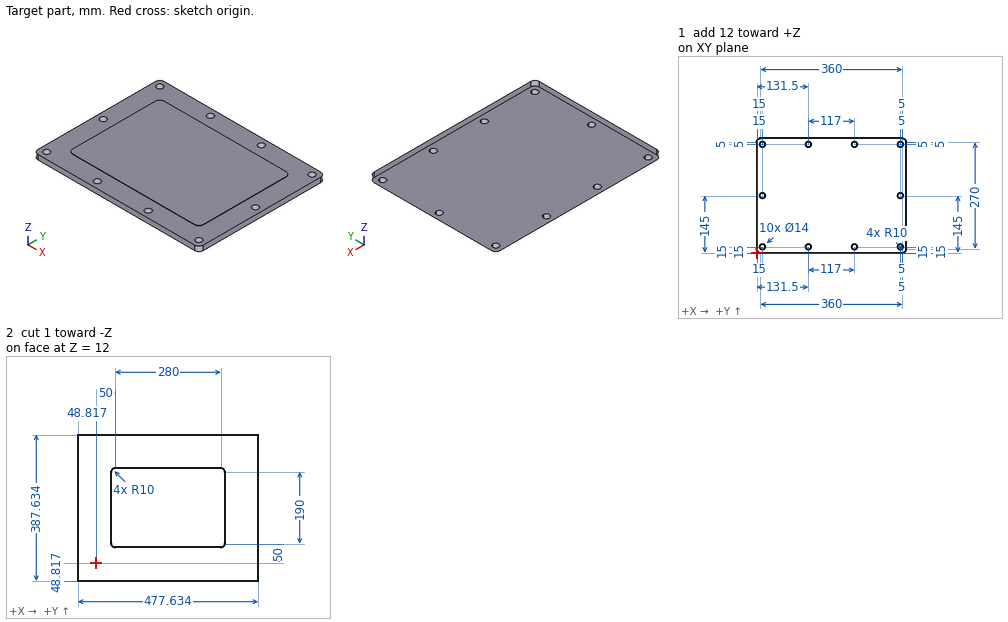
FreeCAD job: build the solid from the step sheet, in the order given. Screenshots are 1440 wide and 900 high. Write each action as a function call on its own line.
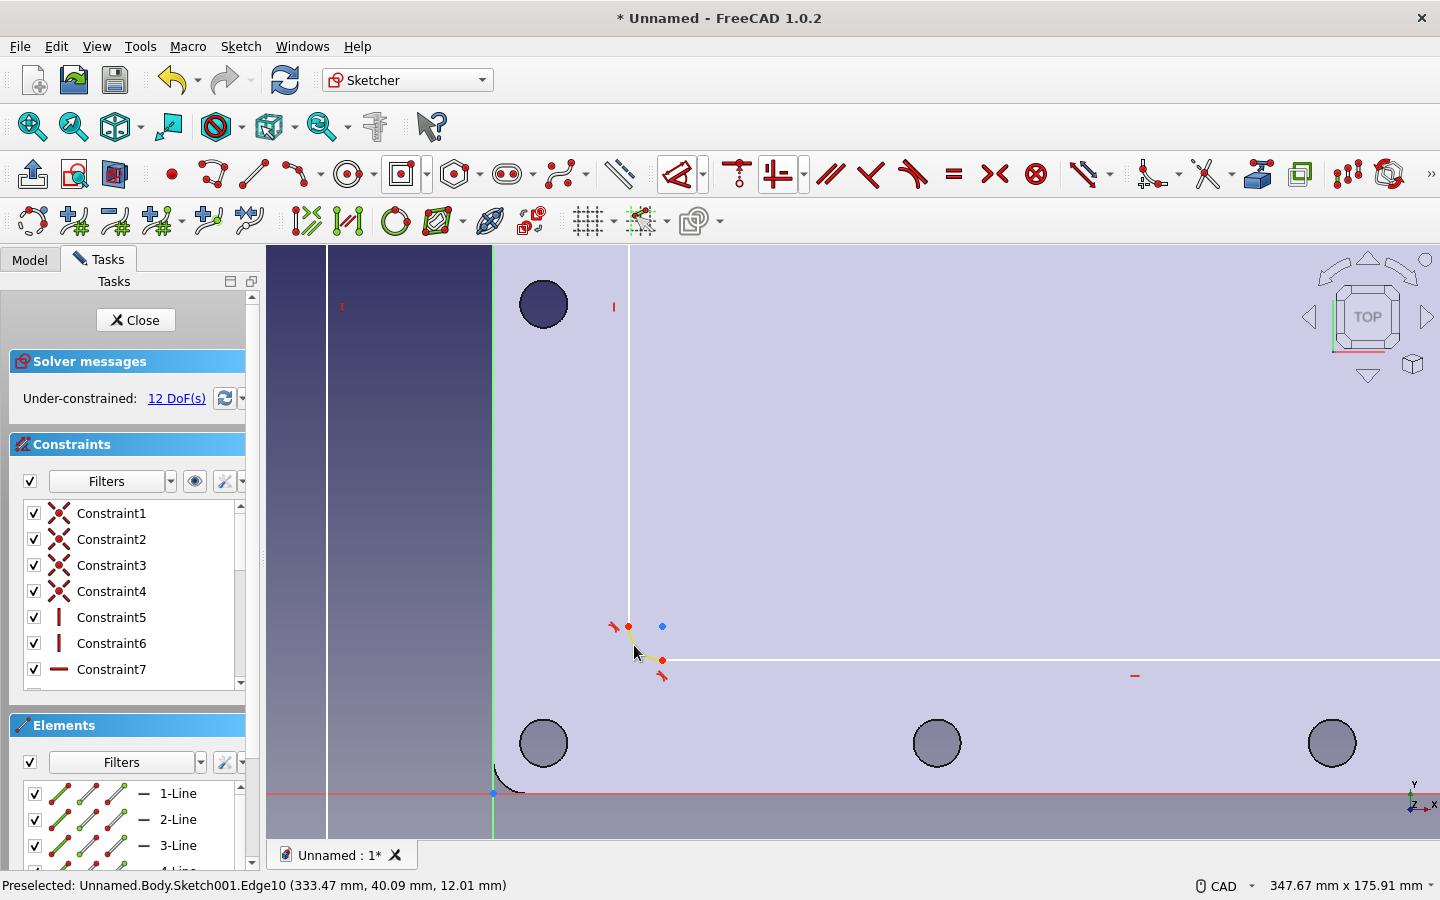
click(633, 642)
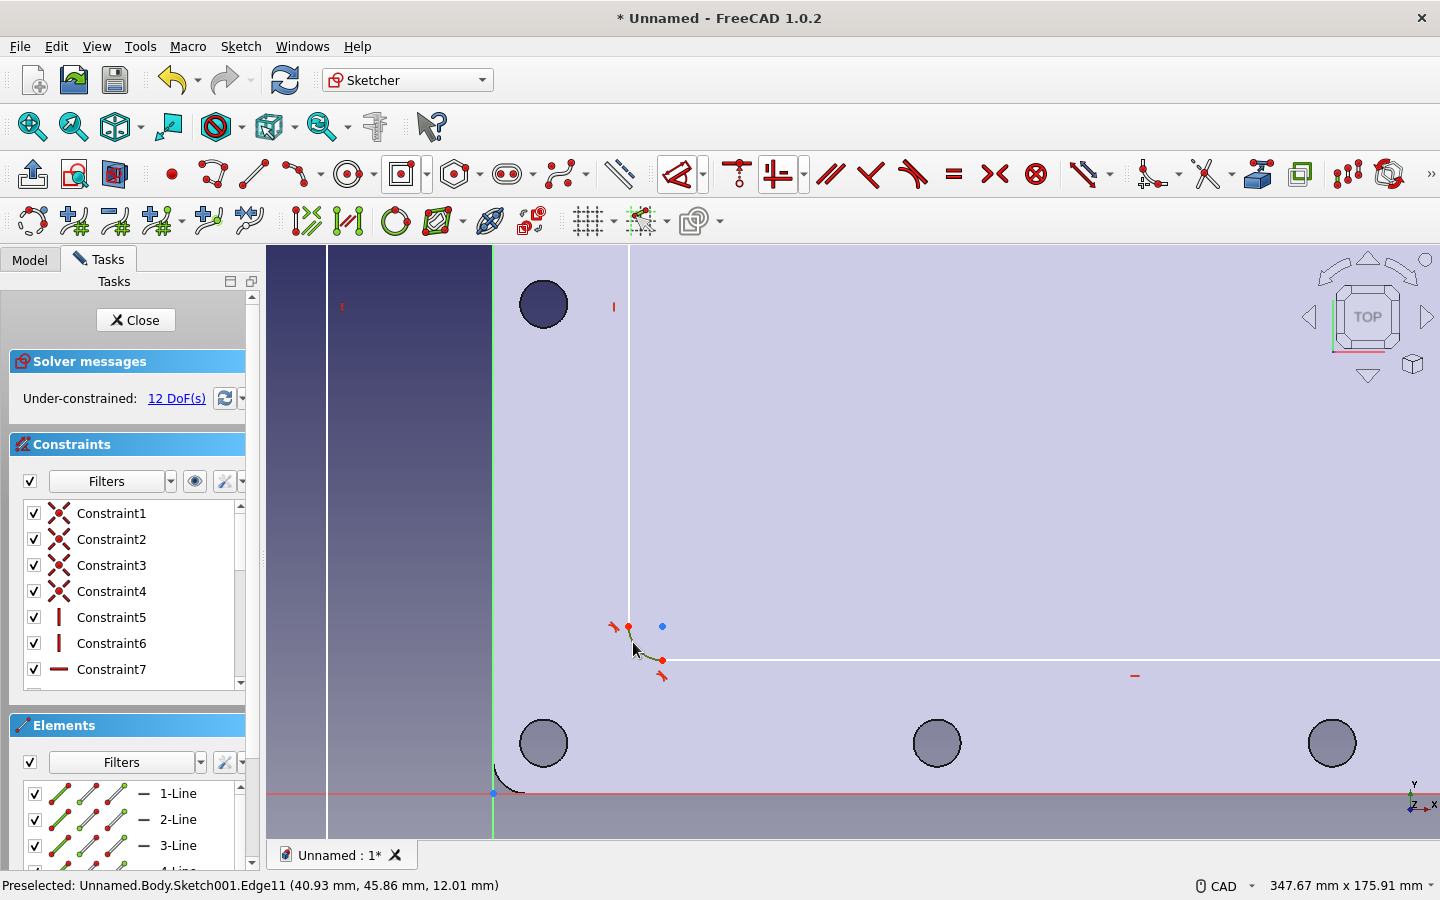
scroll(634, 645, down, 6)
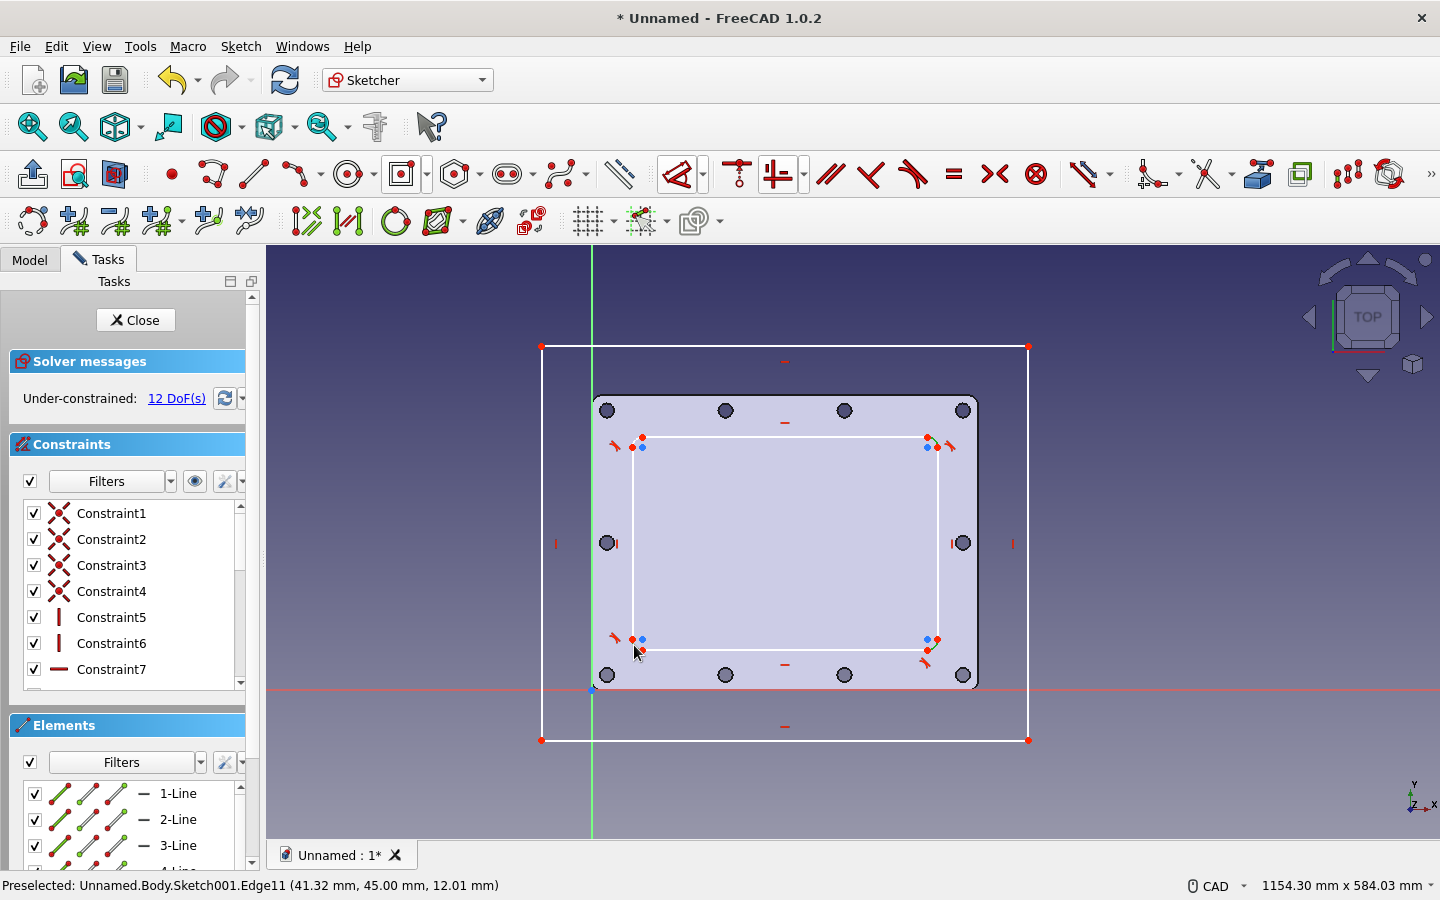
scroll(638, 438, up, 6)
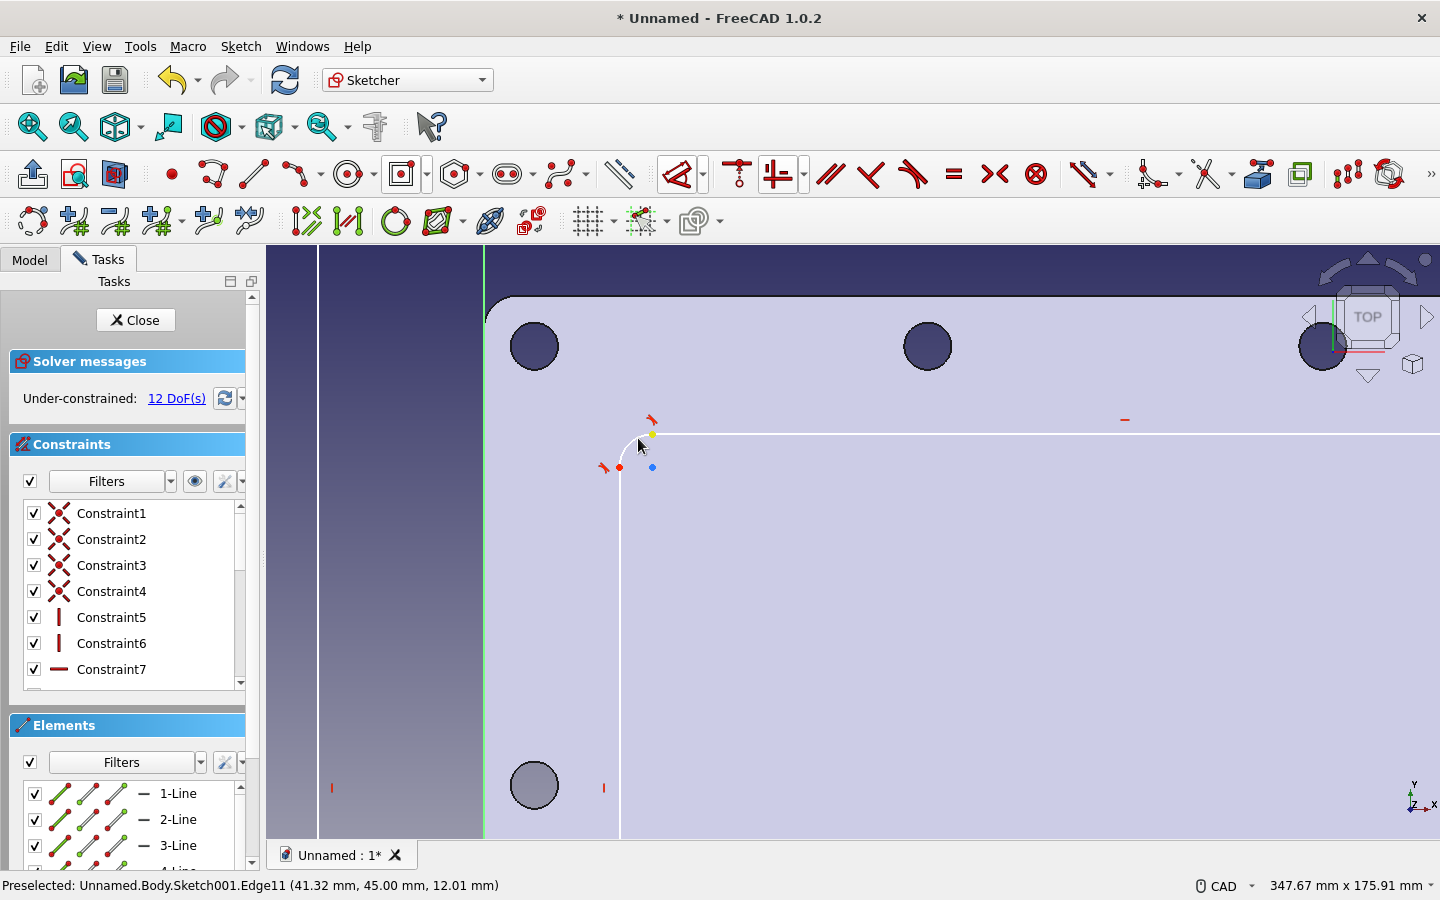
click(637, 438)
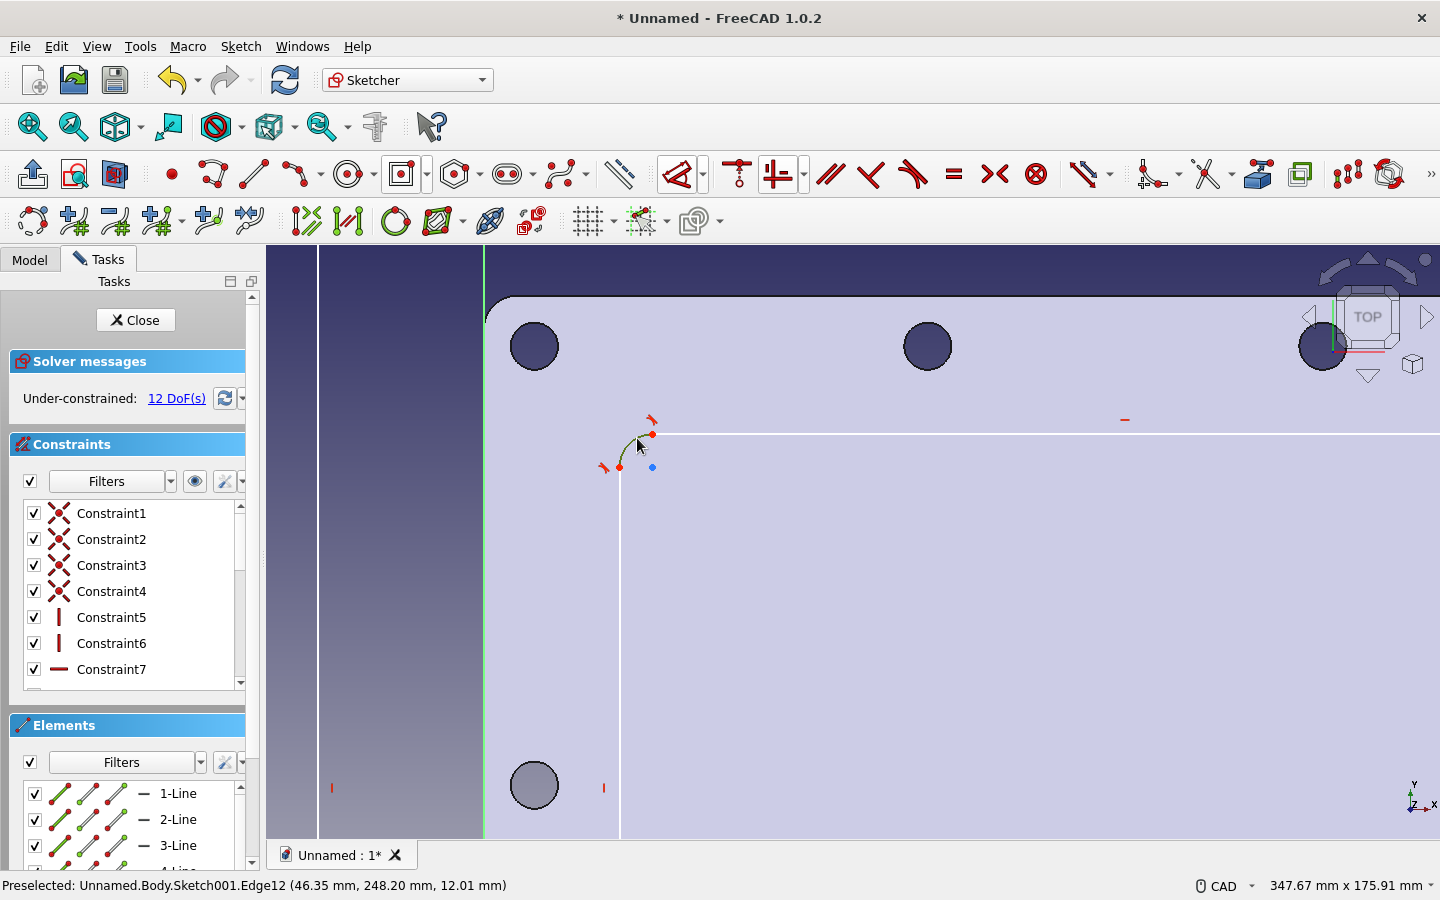
click(954, 174)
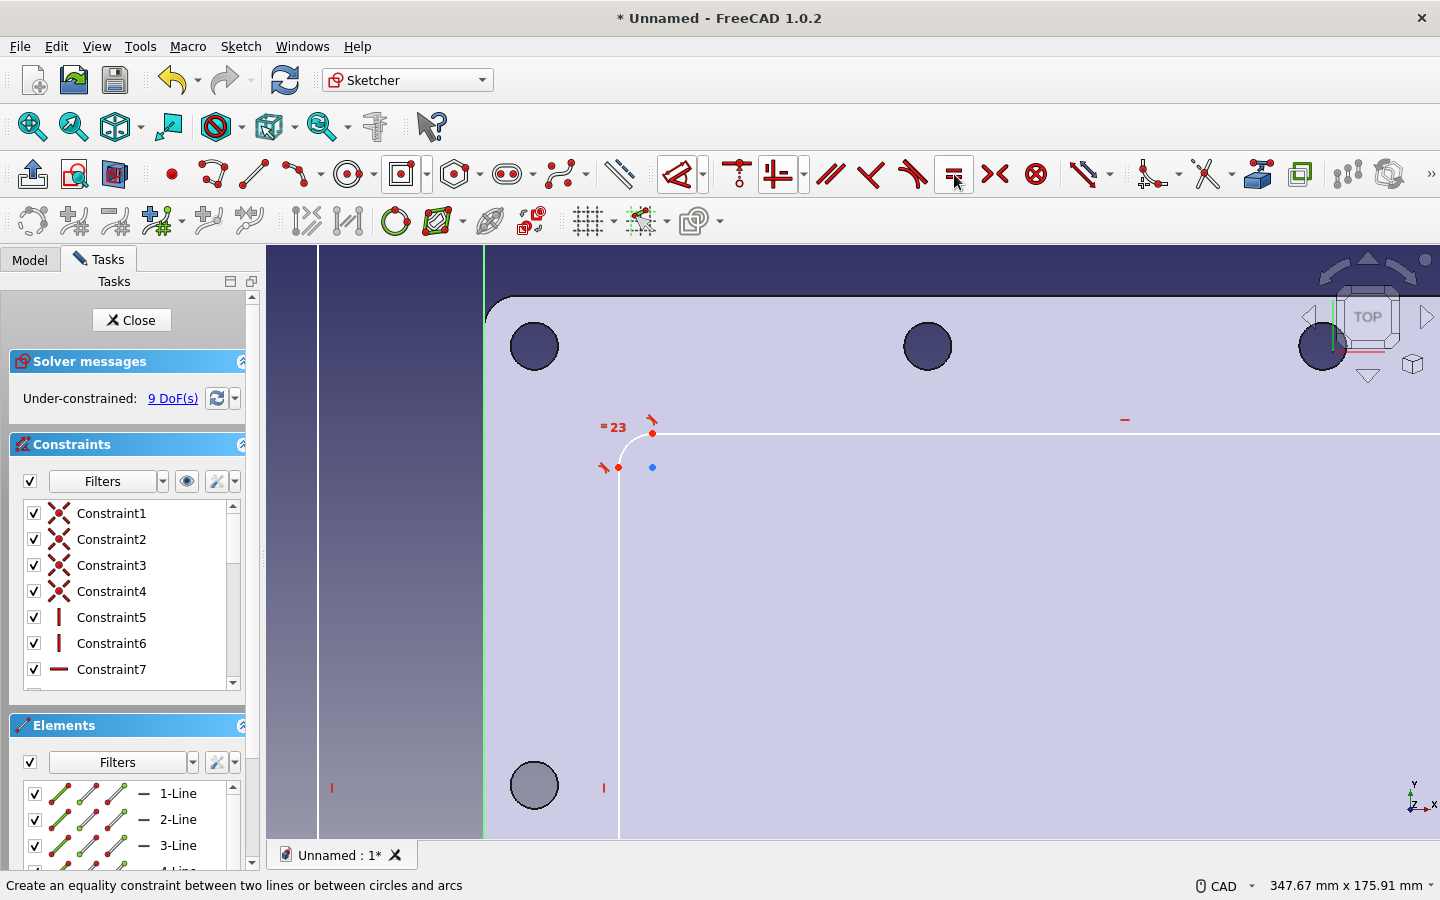
scroll(638, 437, down, 6)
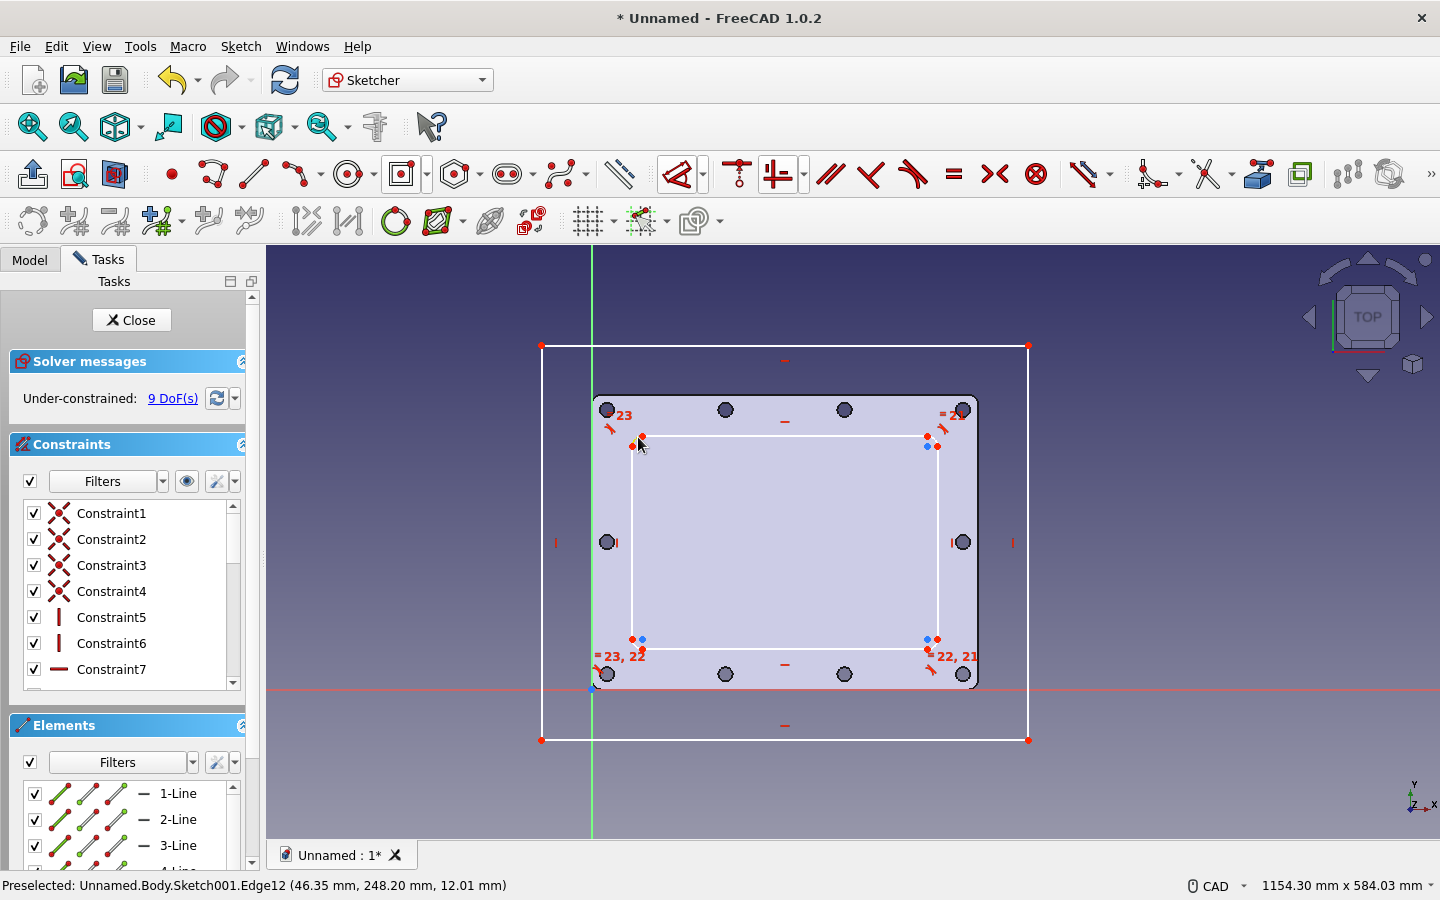
scroll(937, 442, up, 7)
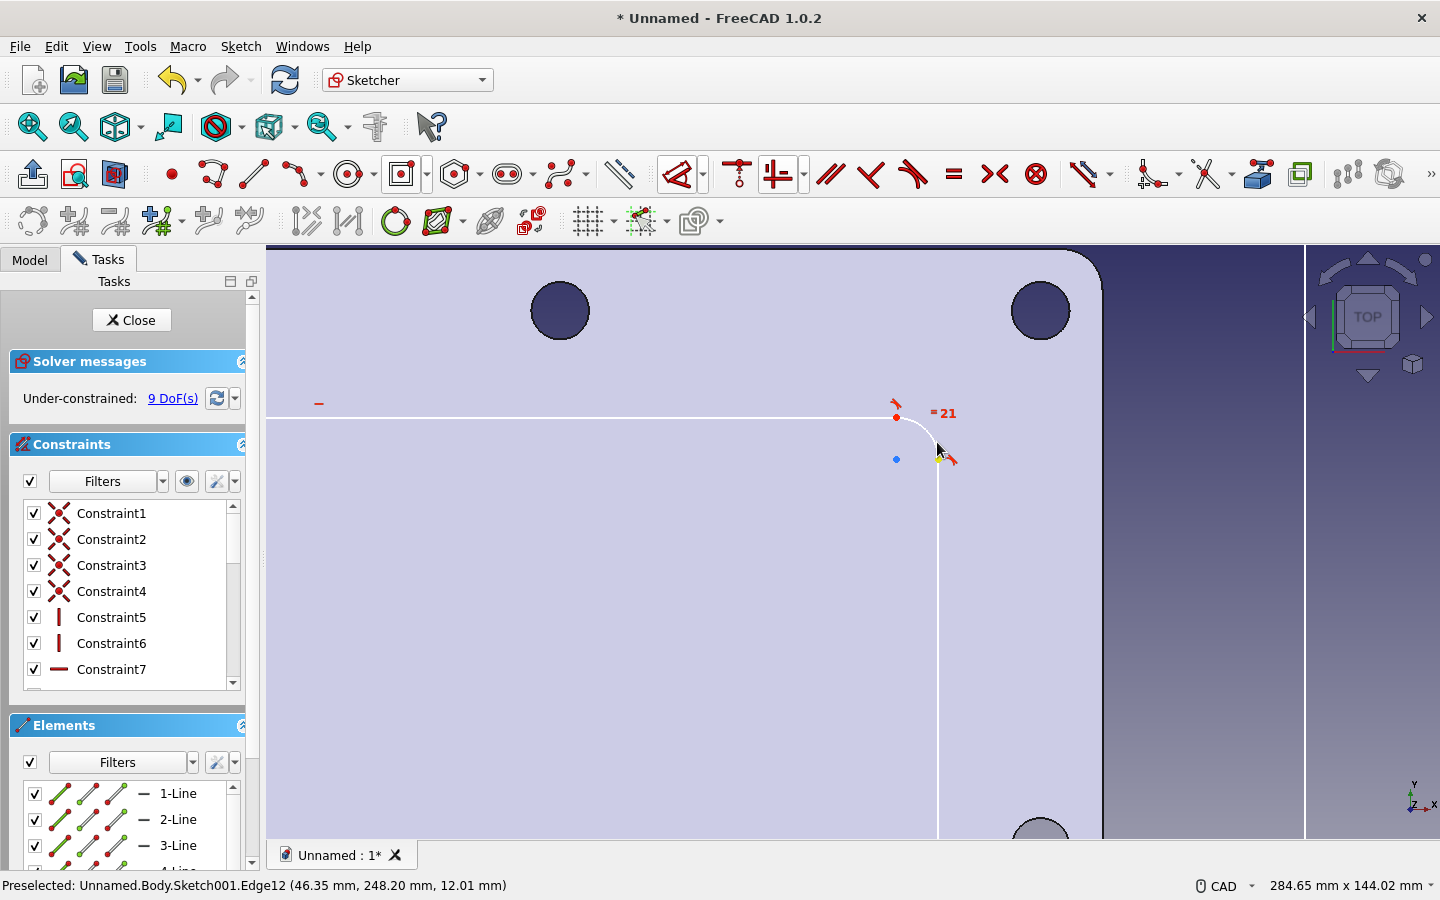
click(934, 440)